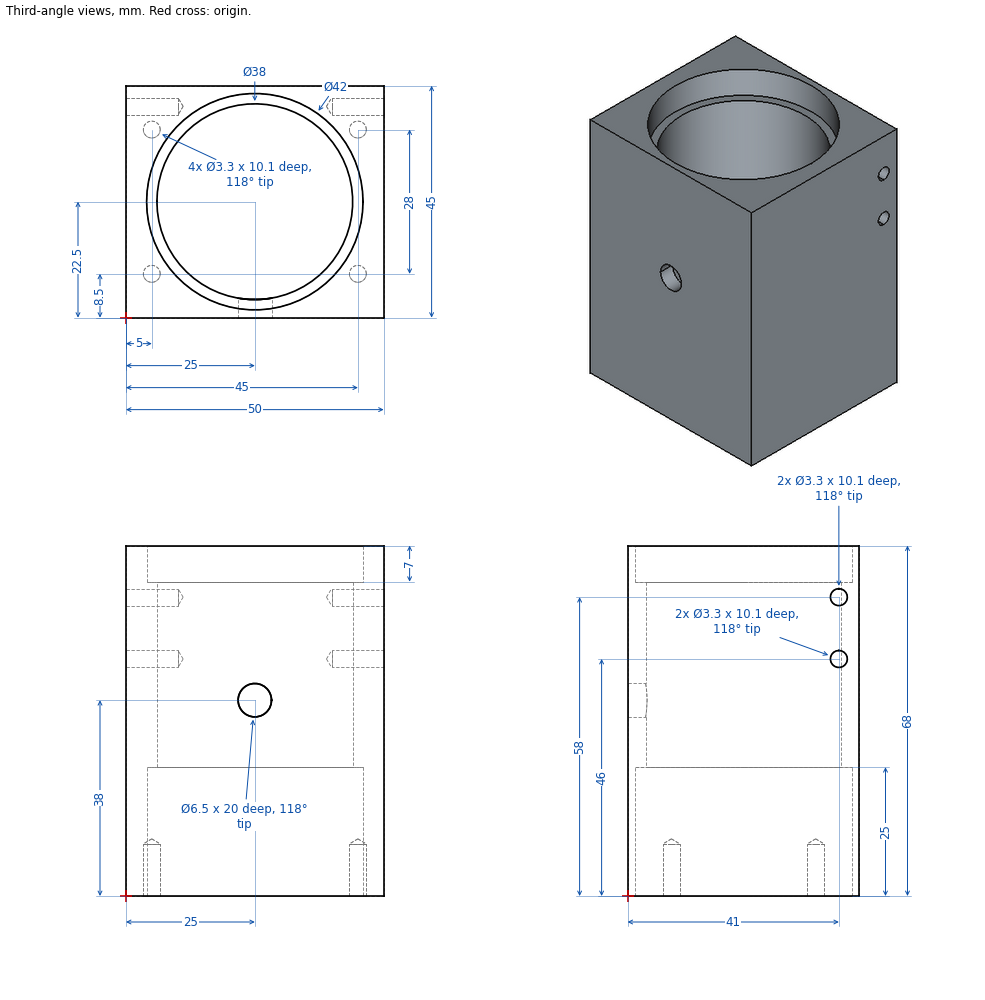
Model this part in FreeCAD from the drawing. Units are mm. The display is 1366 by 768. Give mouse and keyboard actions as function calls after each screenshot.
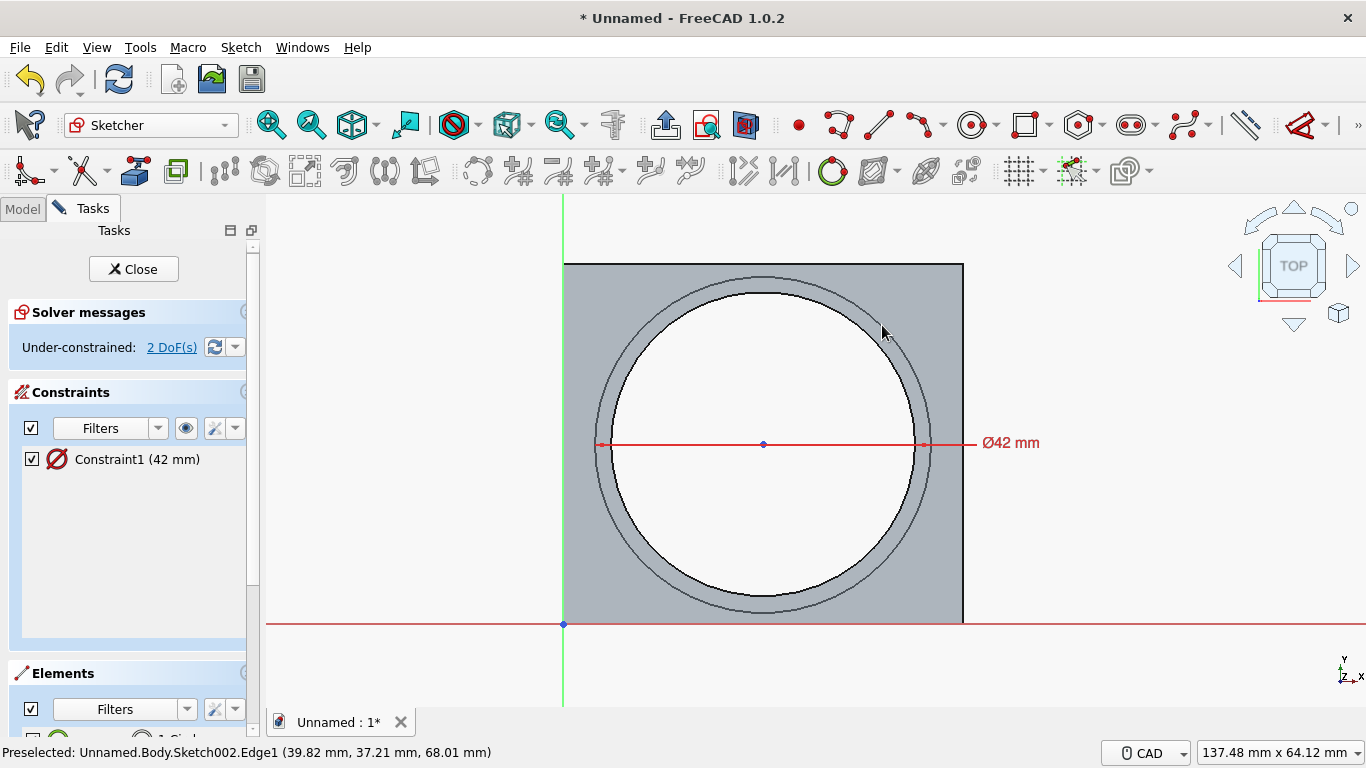
click(1300, 126)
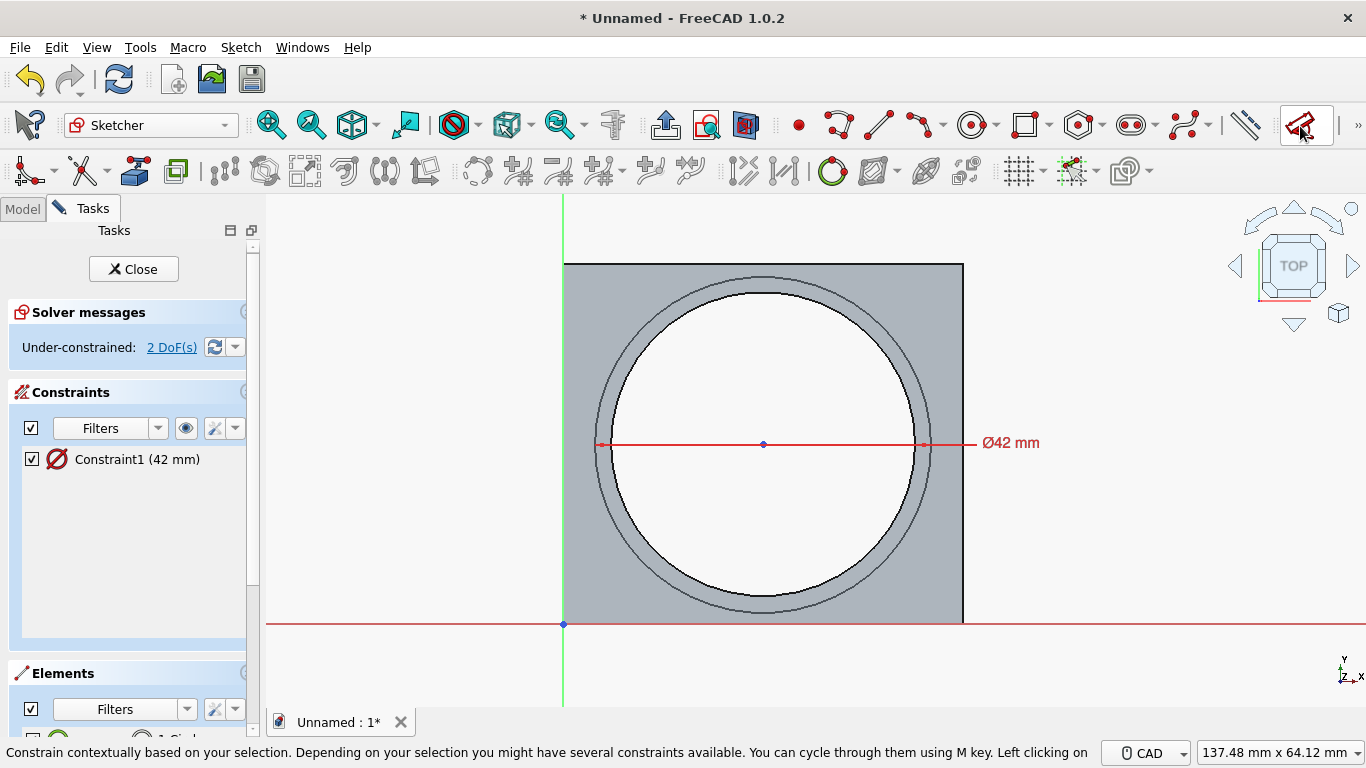
click(763, 445)
click(663, 658)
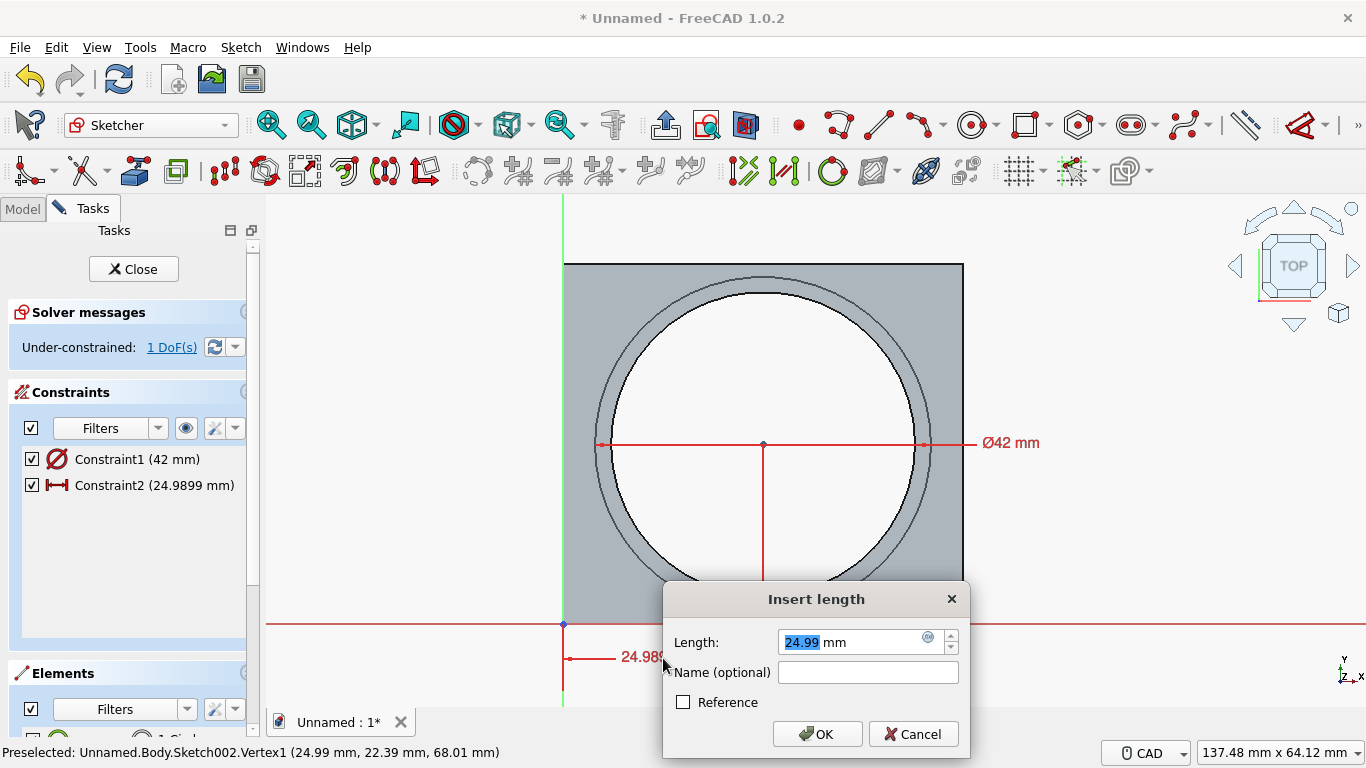
text(25)
key(Return)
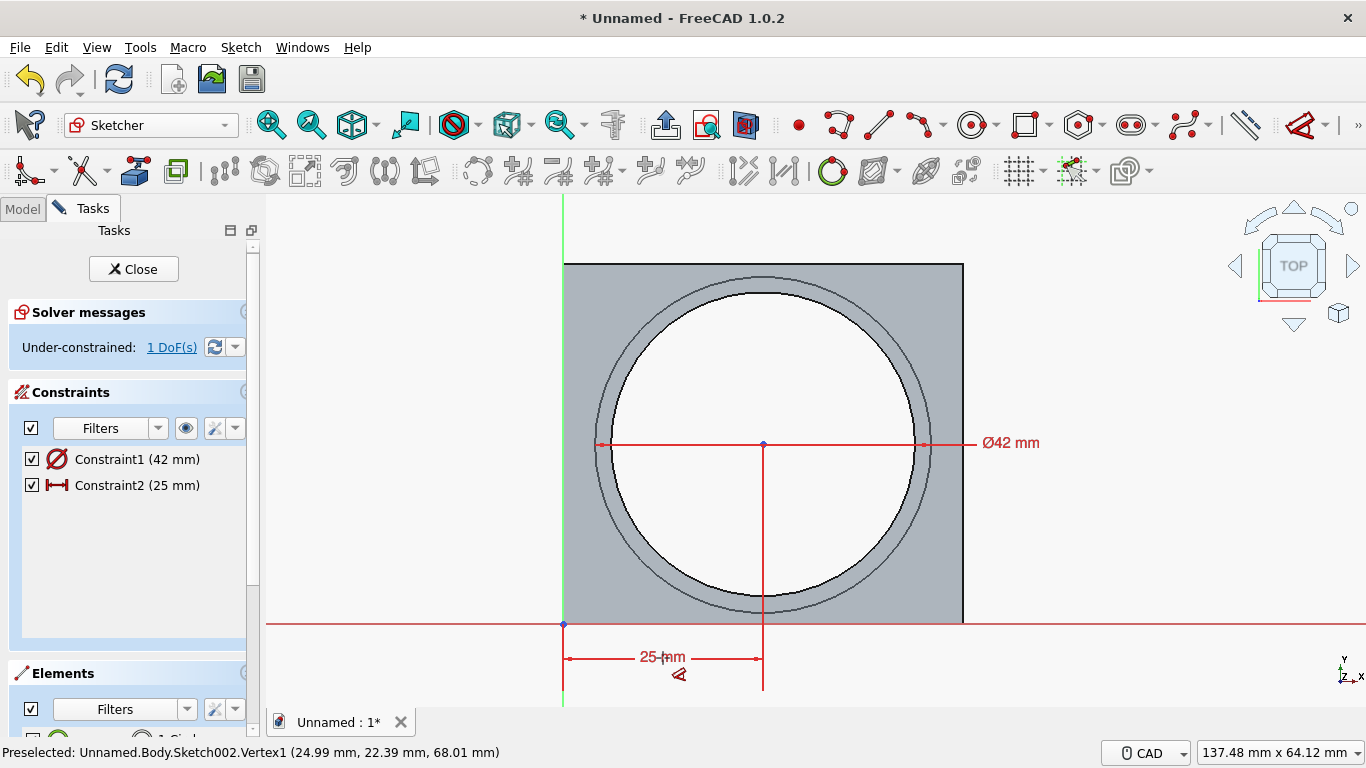
click(763, 445)
click(529, 535)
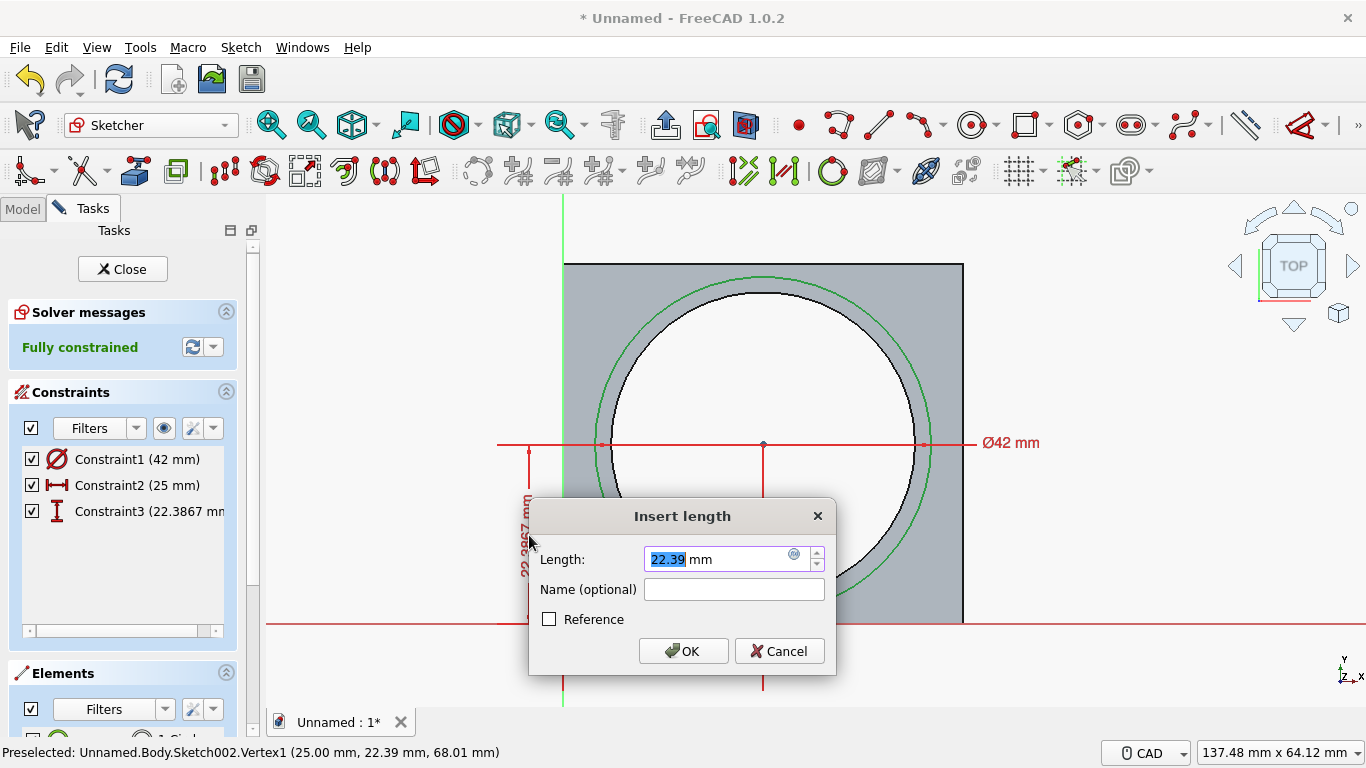
text(22.5)
key(Return)
key(Escape)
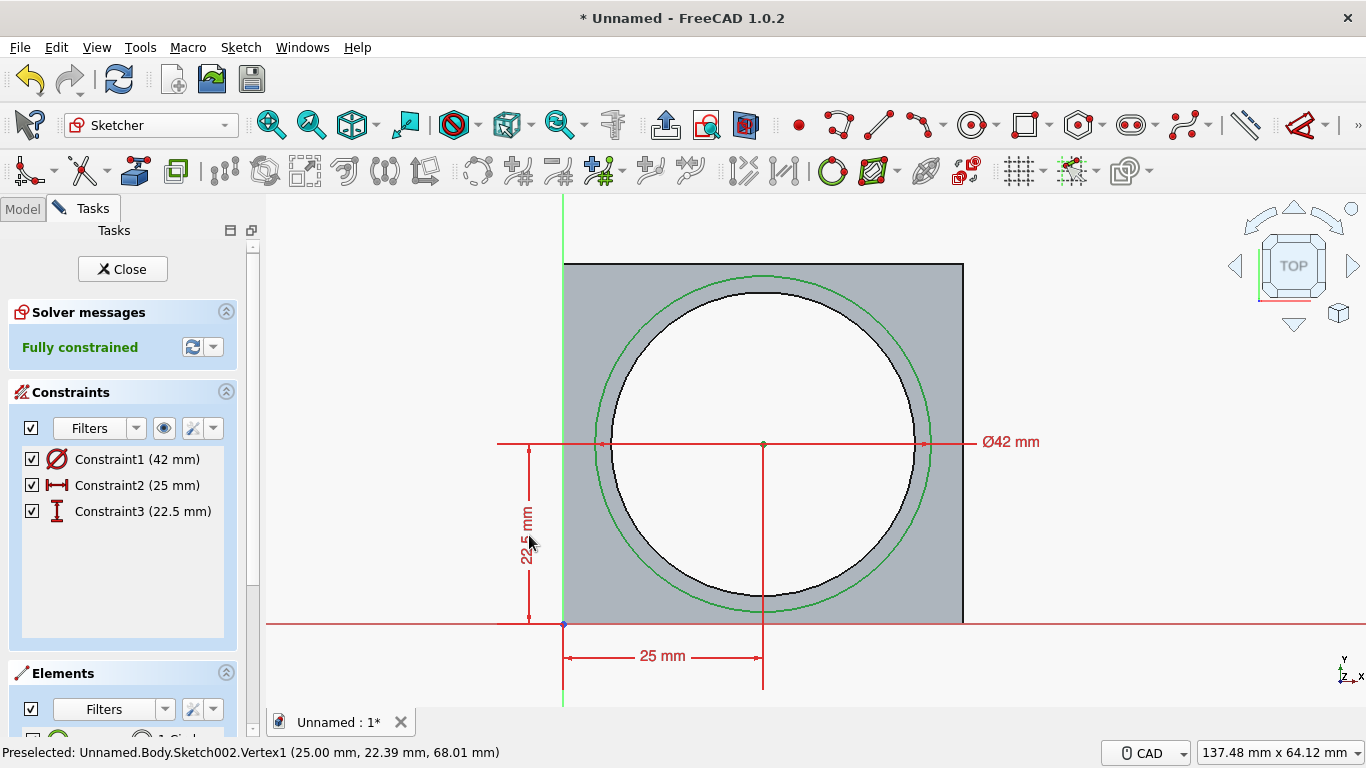
click(123, 269)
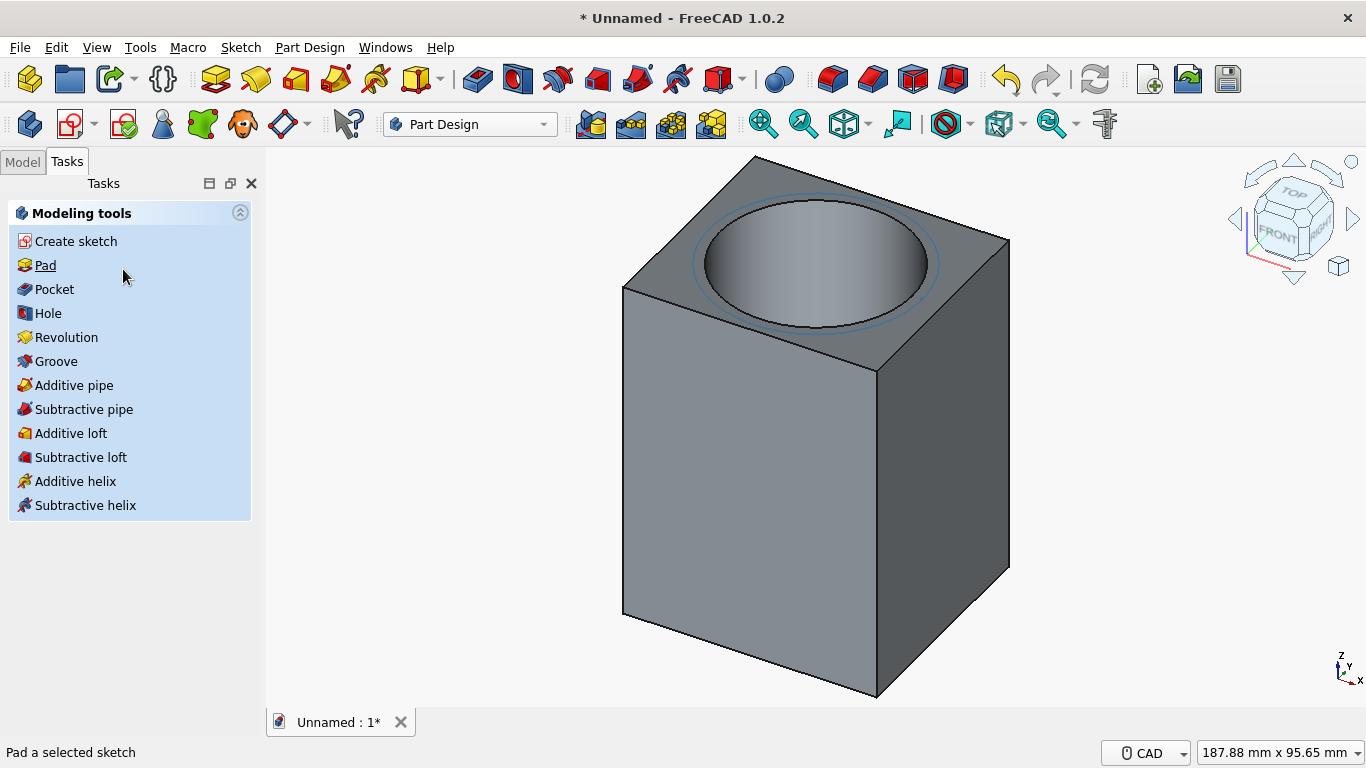
click(478, 80)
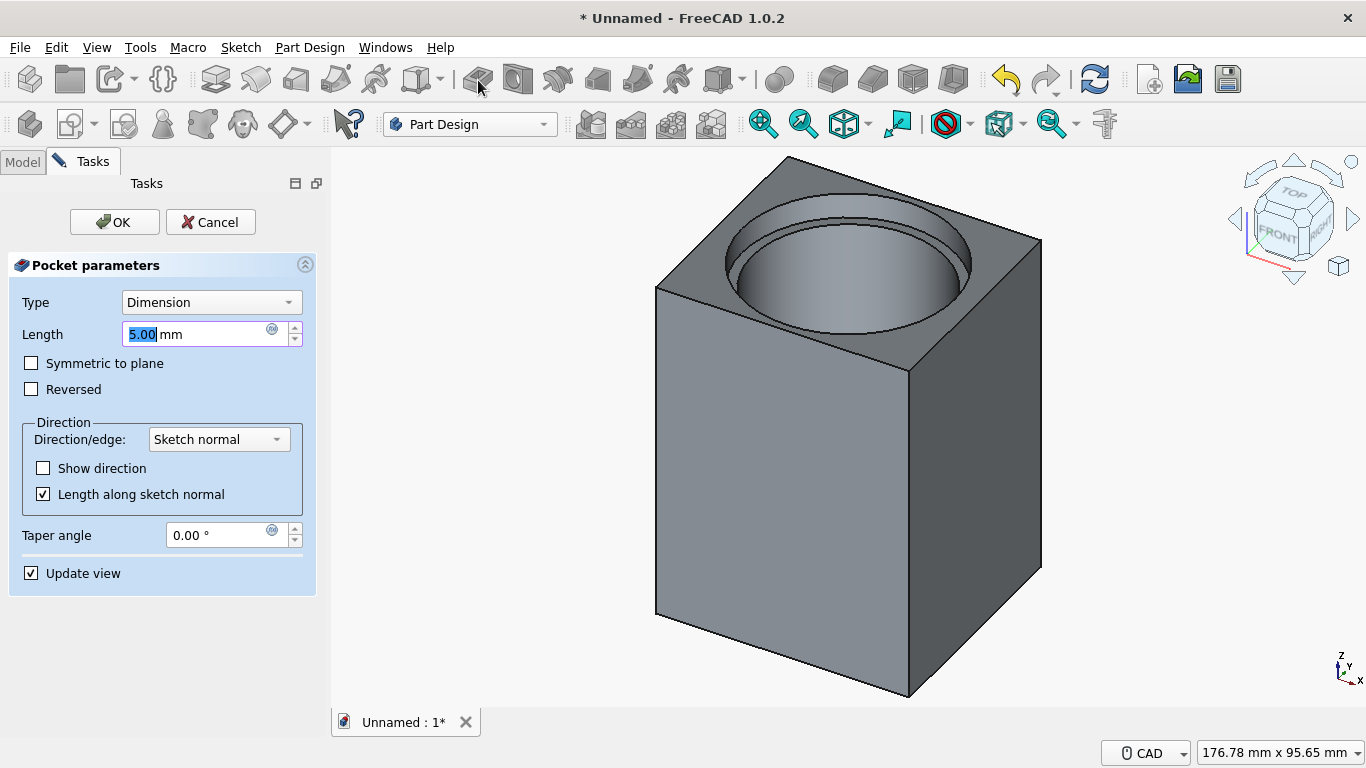
text(7)
key(Tab)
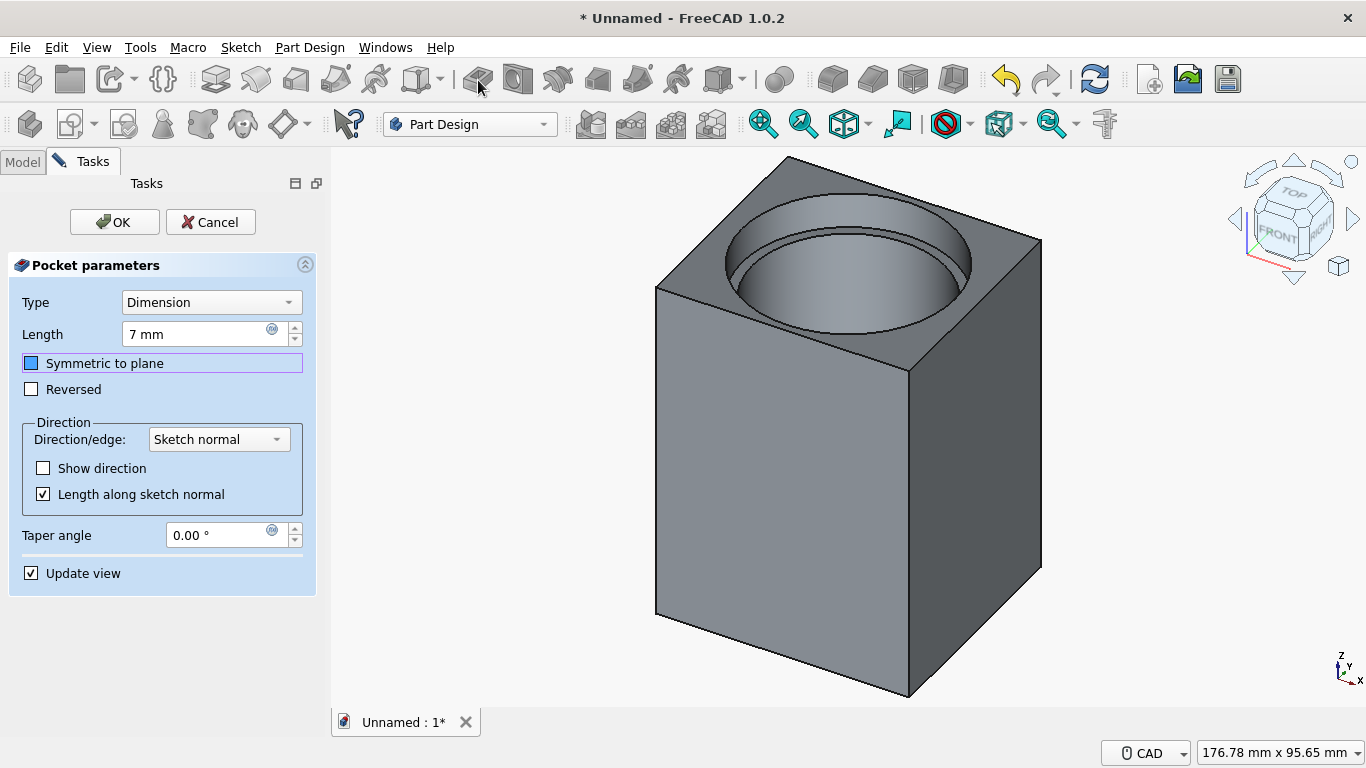
click(115, 222)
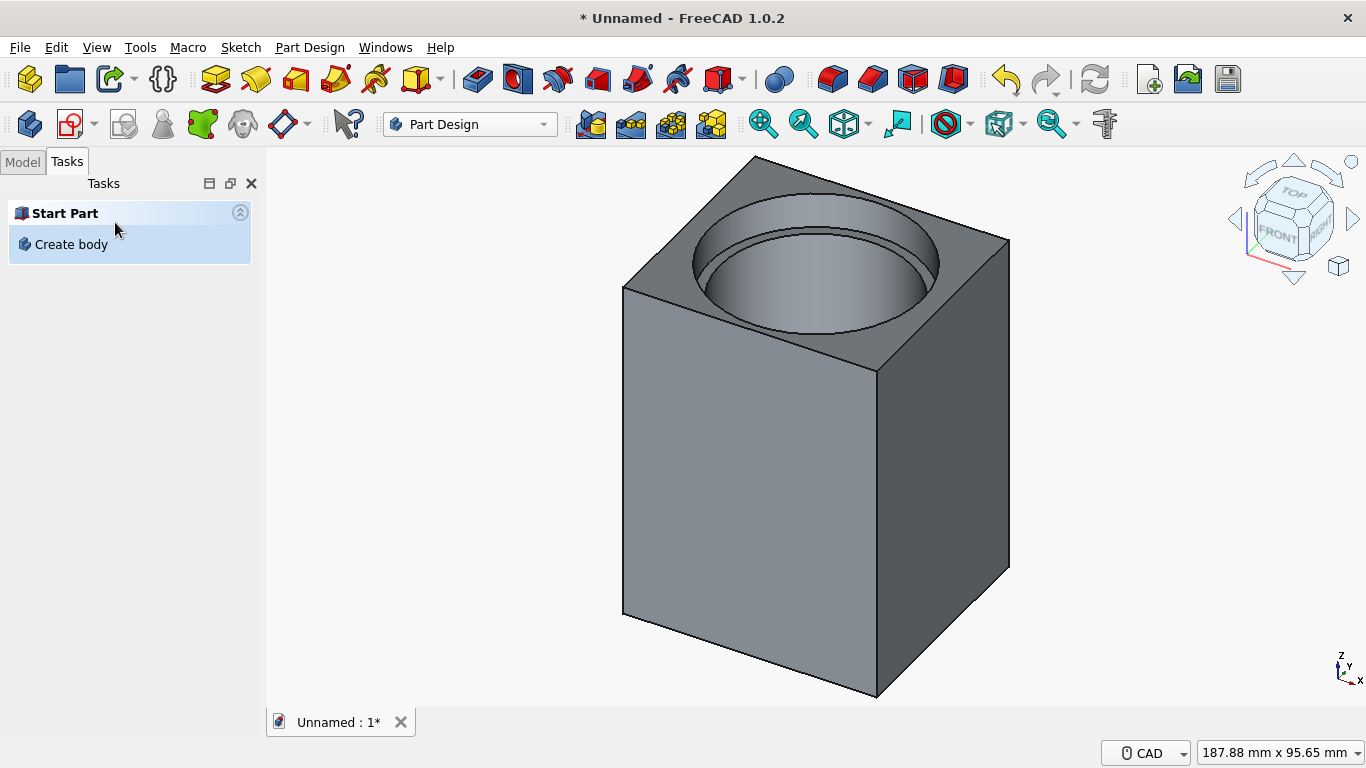
click(23, 161)